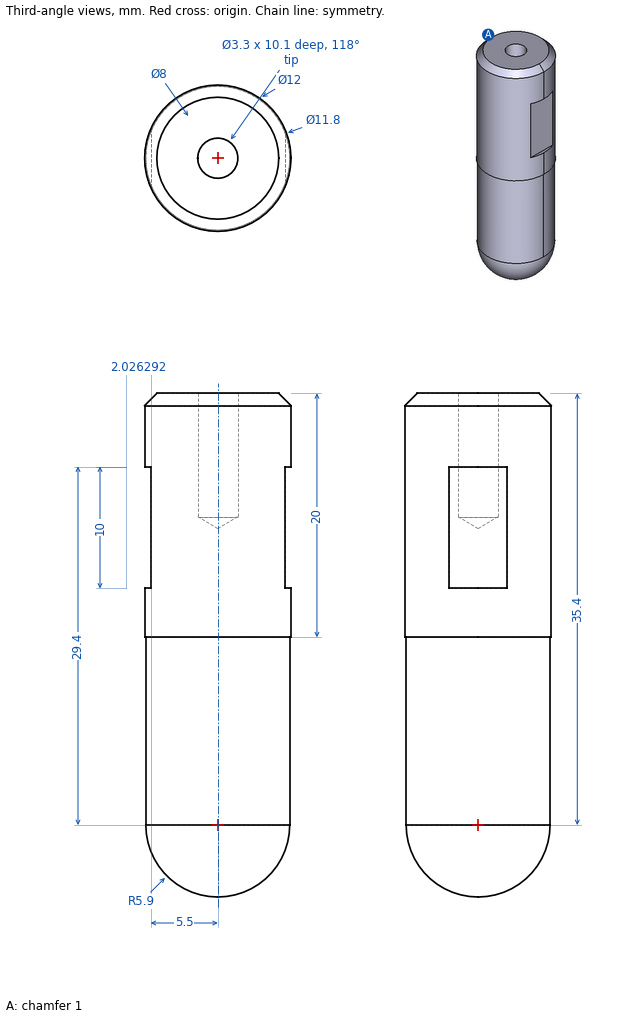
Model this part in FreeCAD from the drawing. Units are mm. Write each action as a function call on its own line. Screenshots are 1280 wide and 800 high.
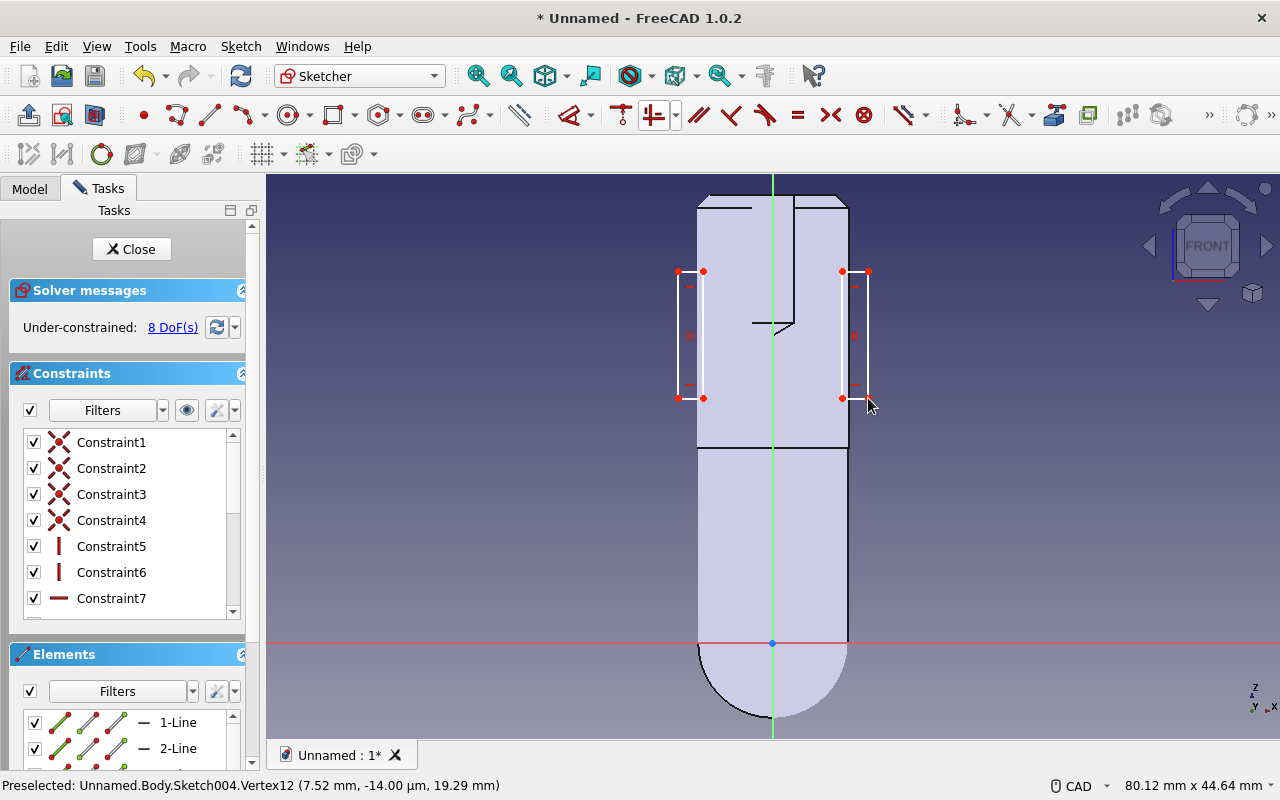
click(703, 272)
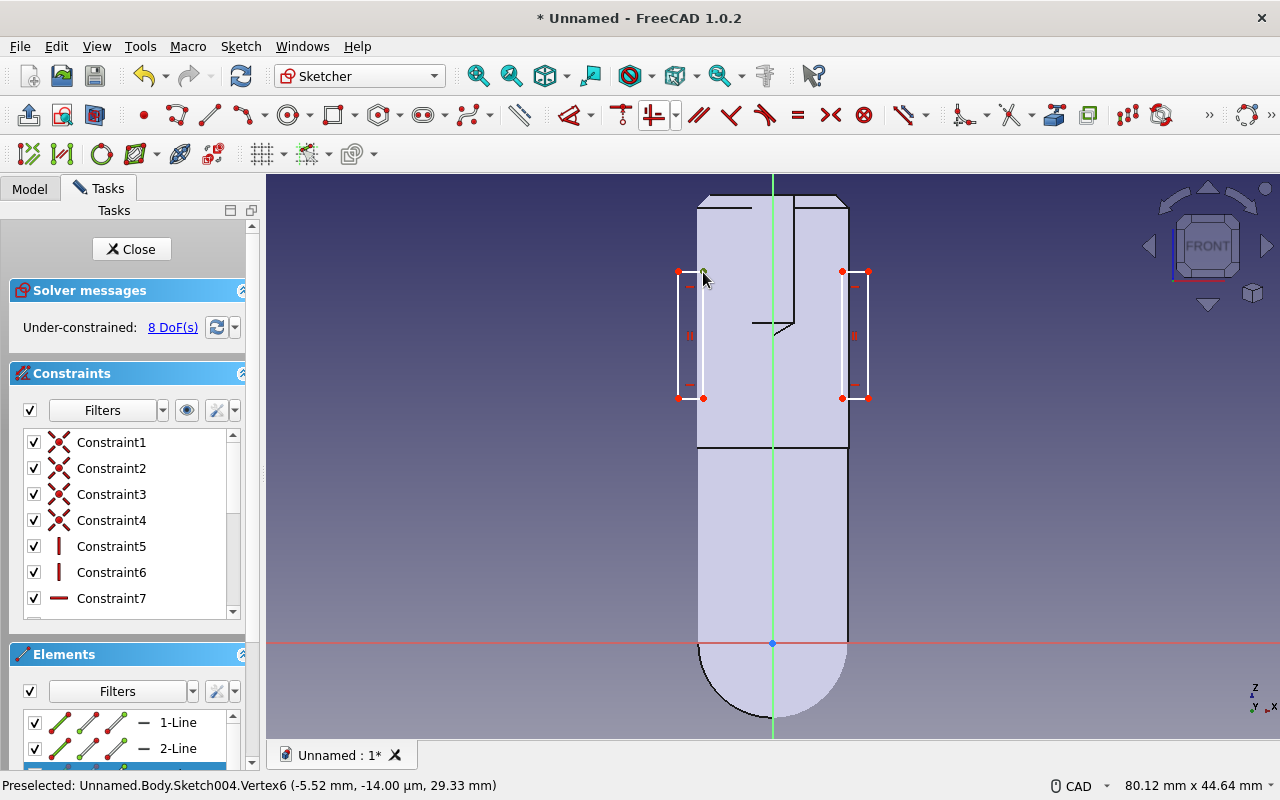
click(842, 272)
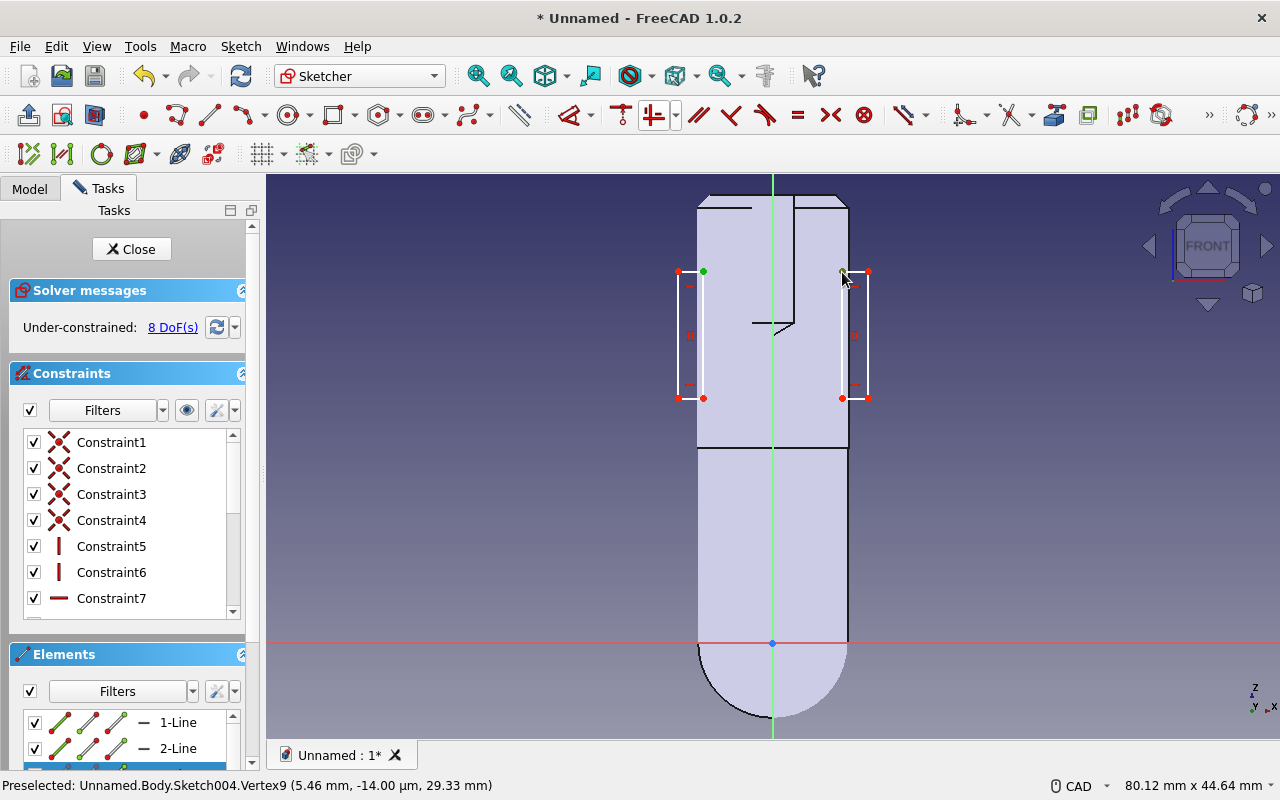
click(773, 675)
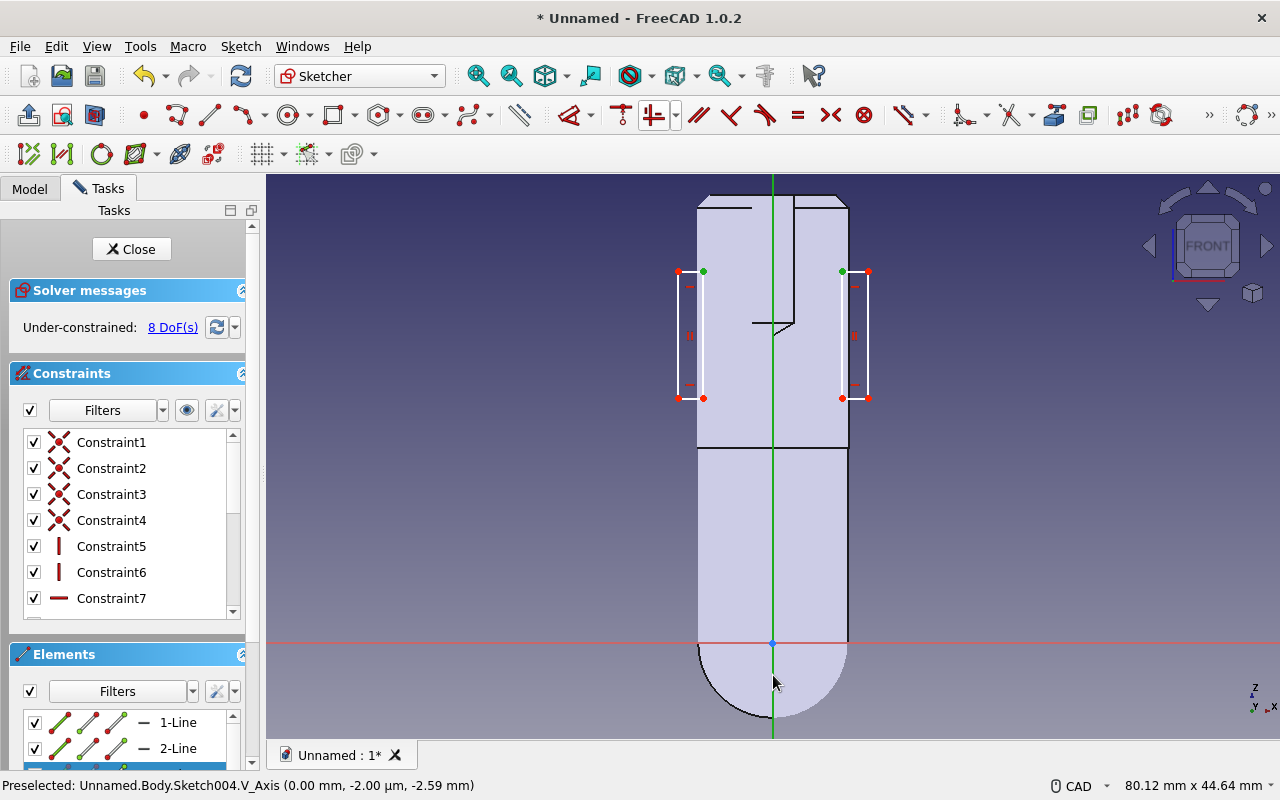
click(831, 116)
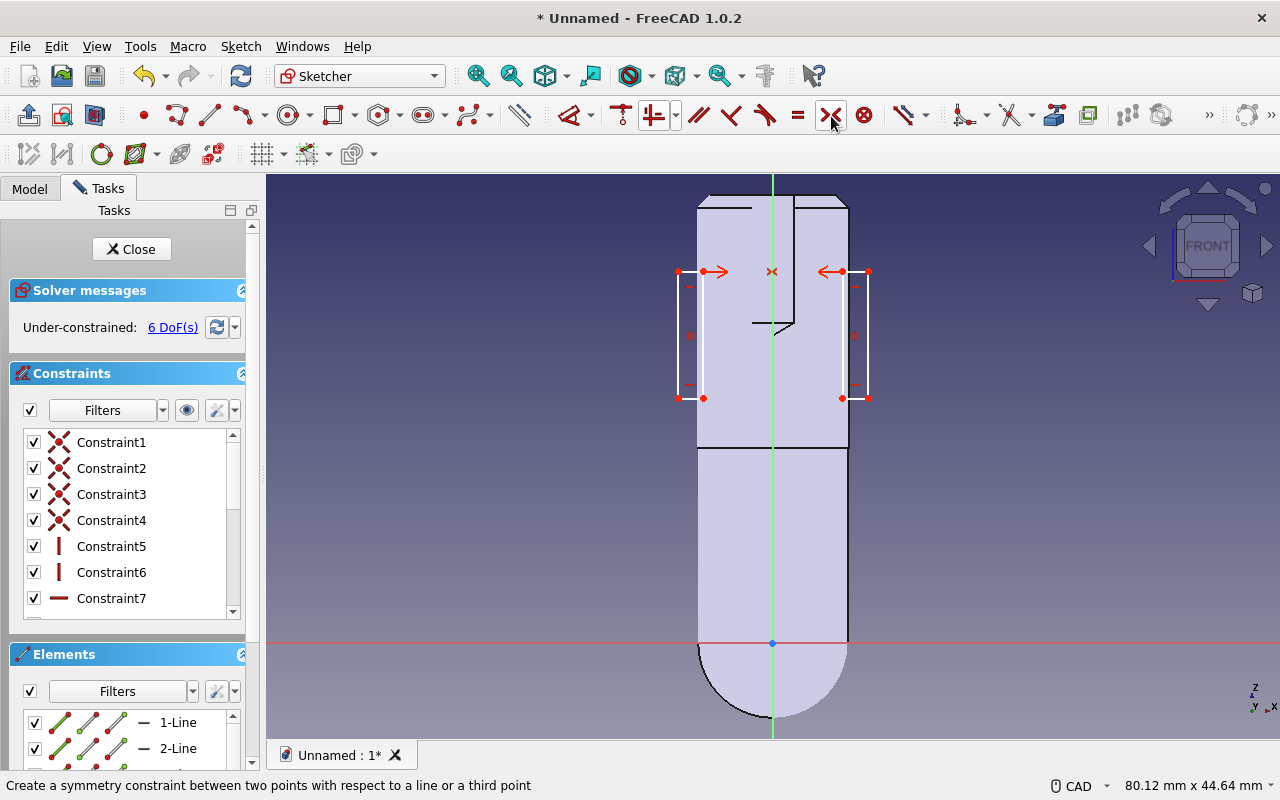
click(678, 399)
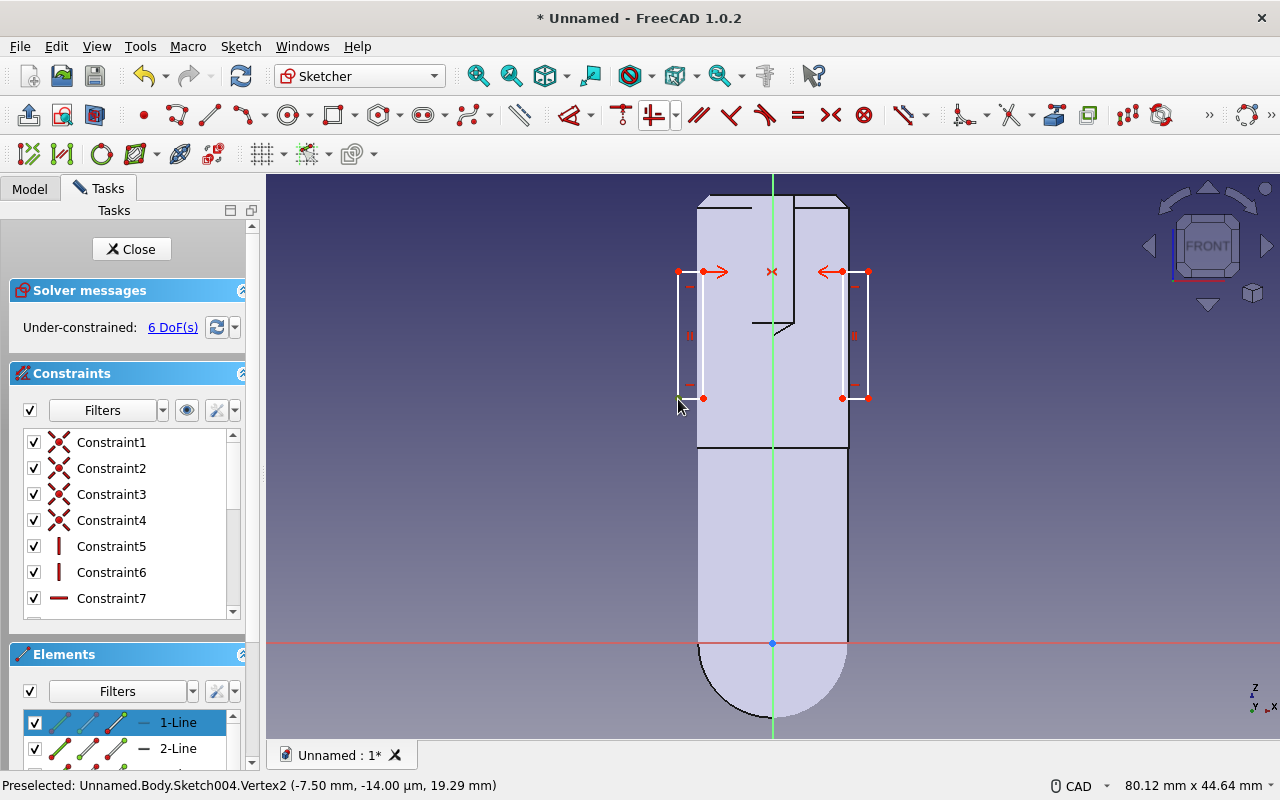
click(868, 399)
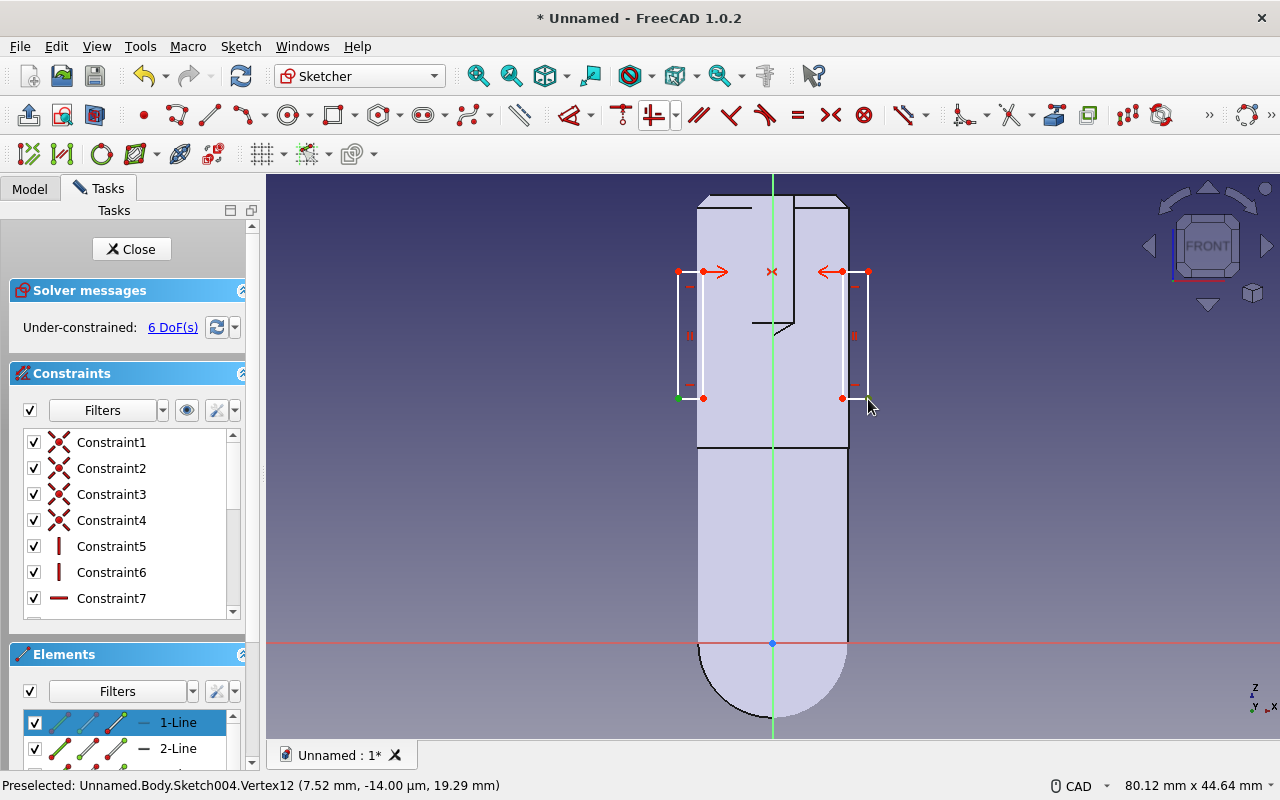
click(773, 675)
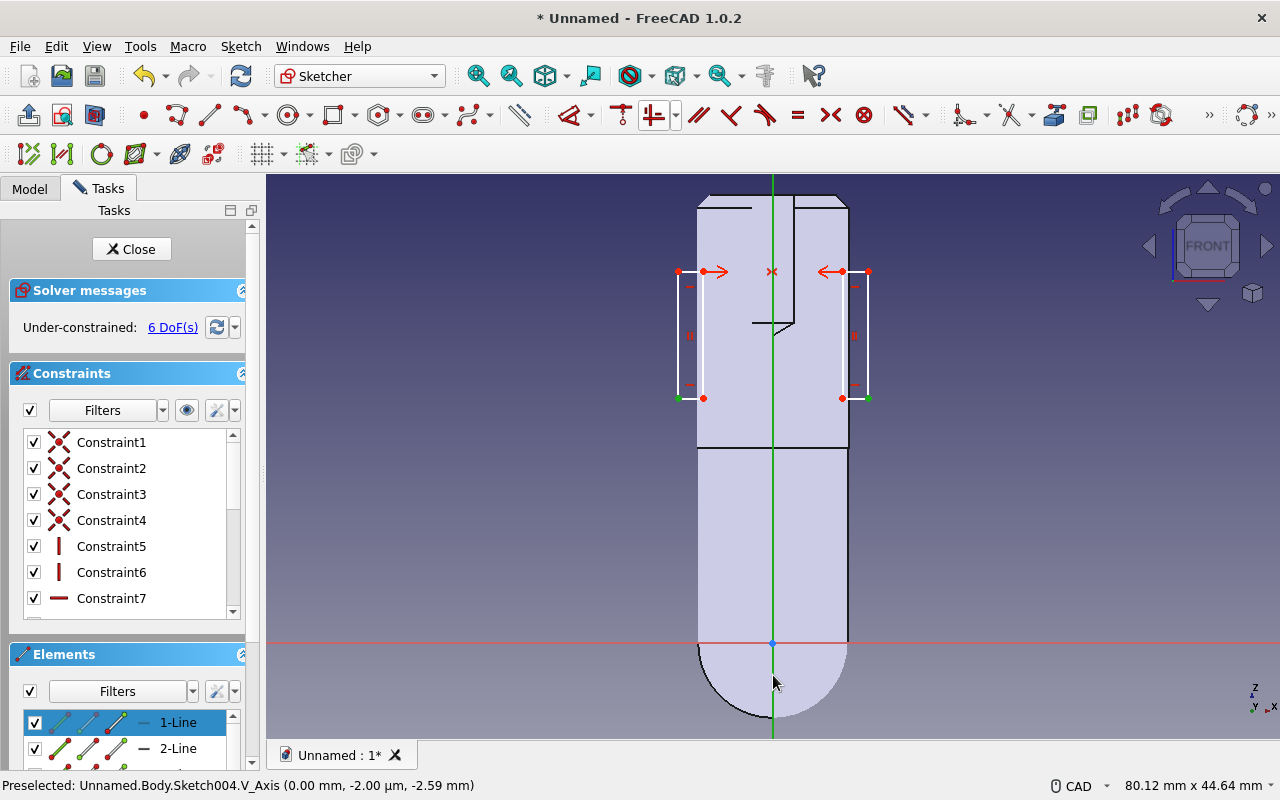
click(831, 116)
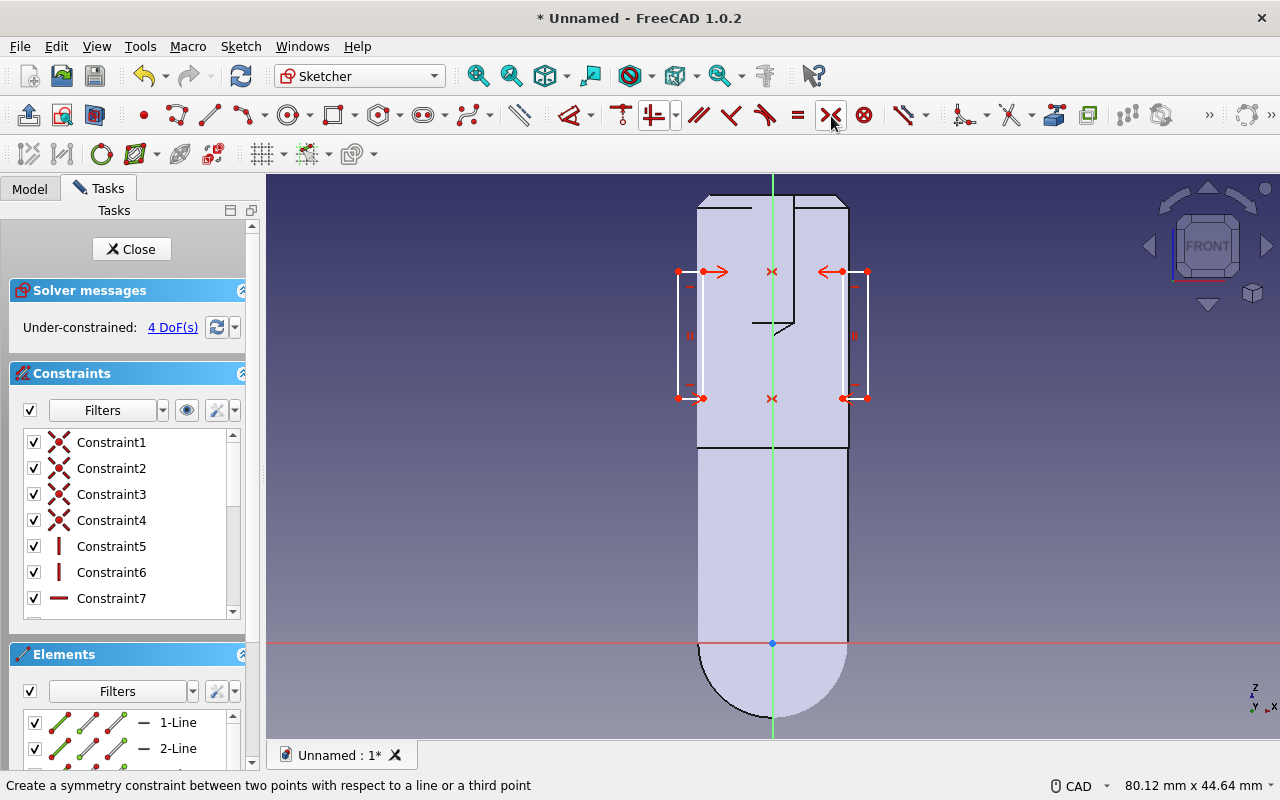
click(568, 116)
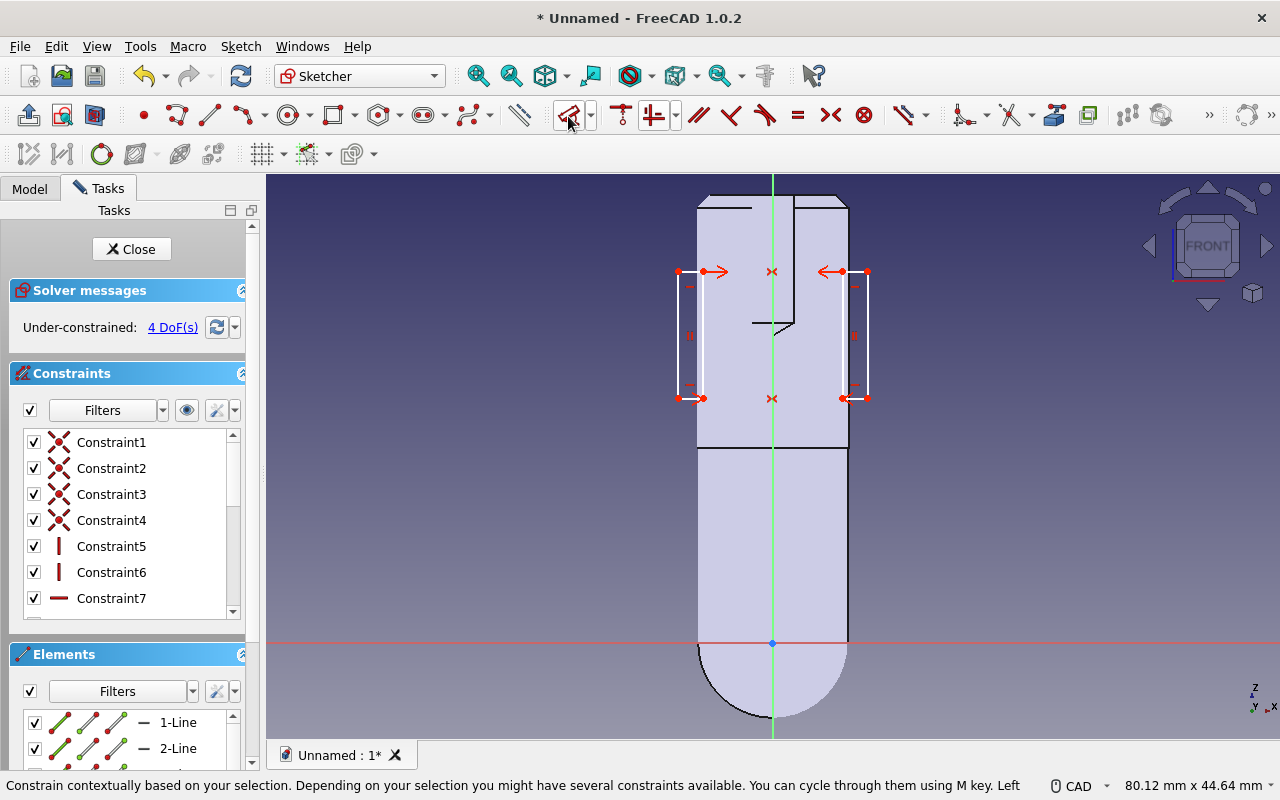
click(678, 310)
click(644, 335)